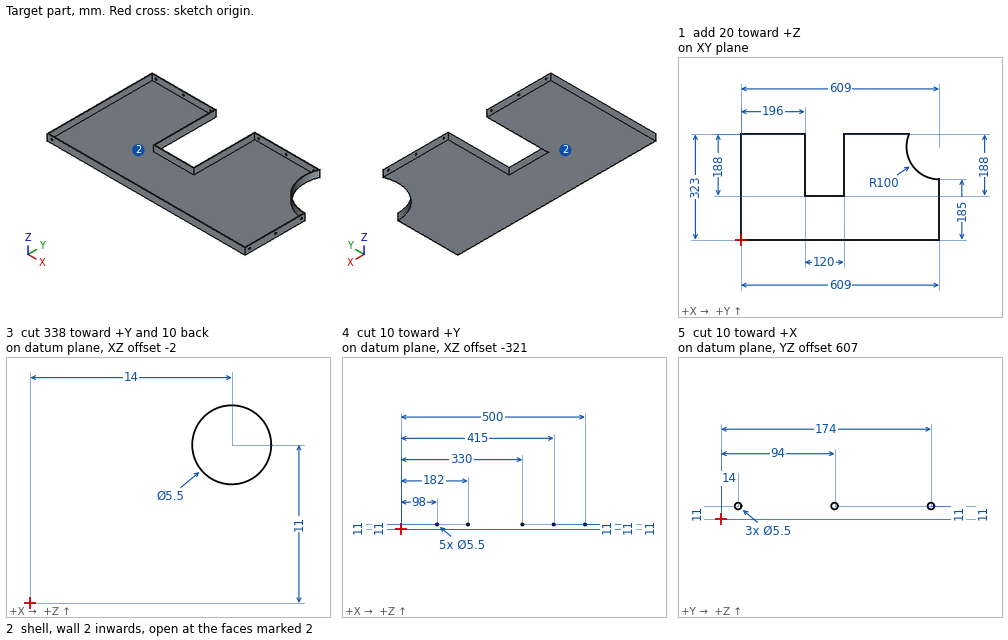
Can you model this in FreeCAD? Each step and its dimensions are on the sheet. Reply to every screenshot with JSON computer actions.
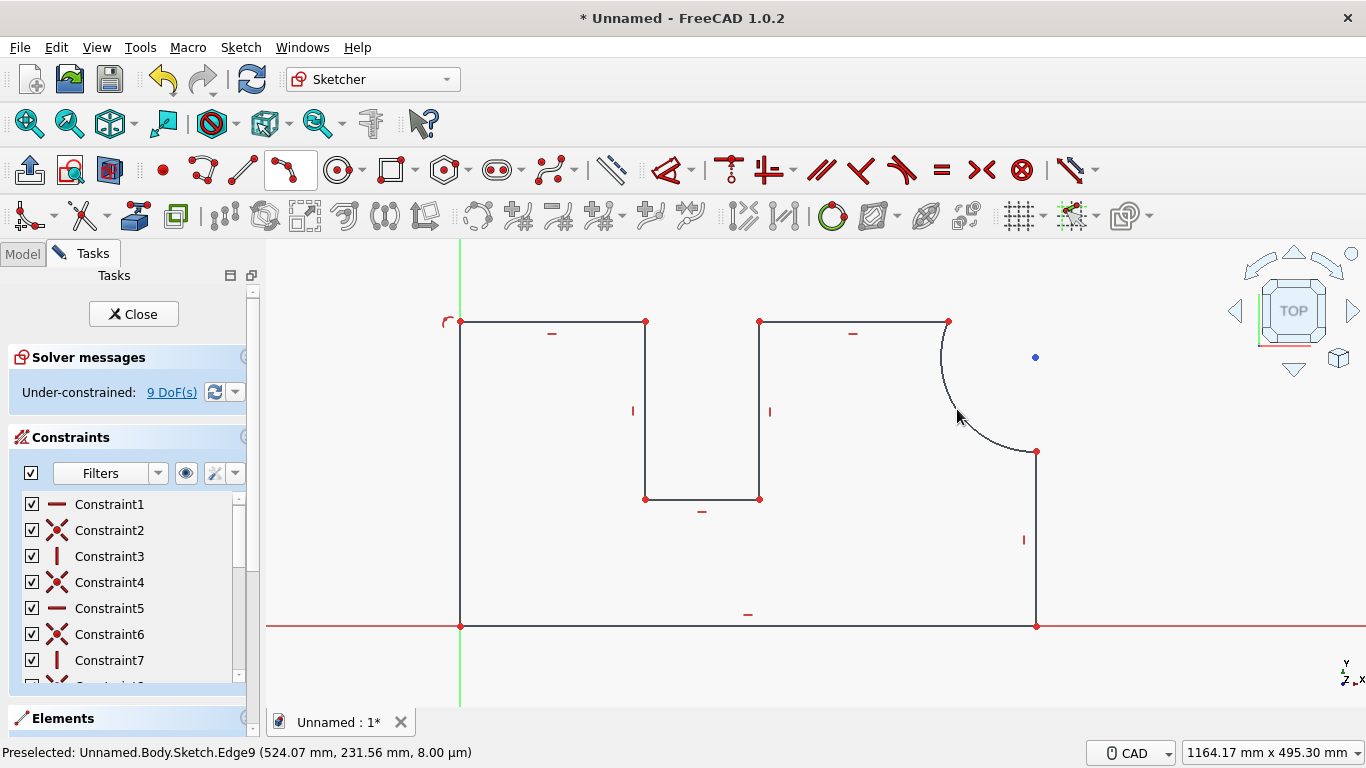
{"action": "left_click", "coordinate": [943, 377]}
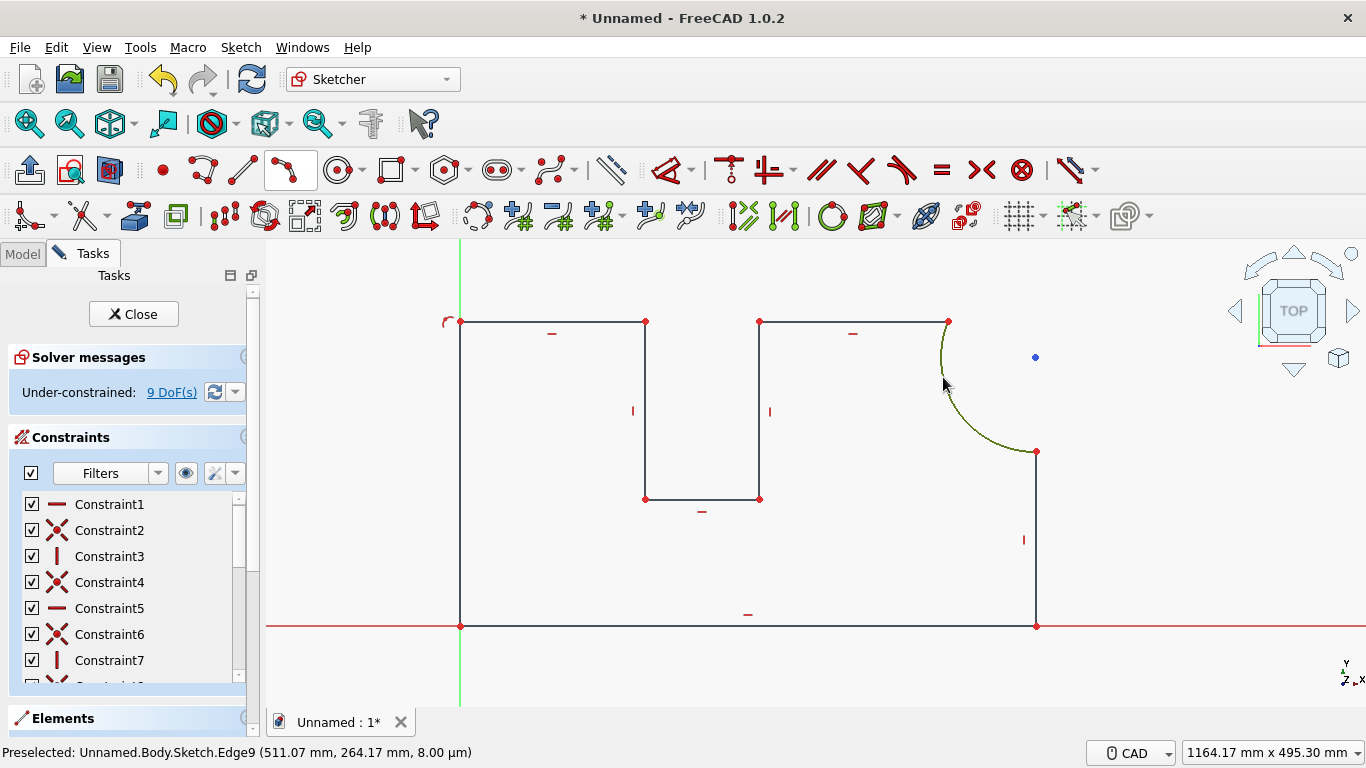
{"action": "key", "text": "k r"}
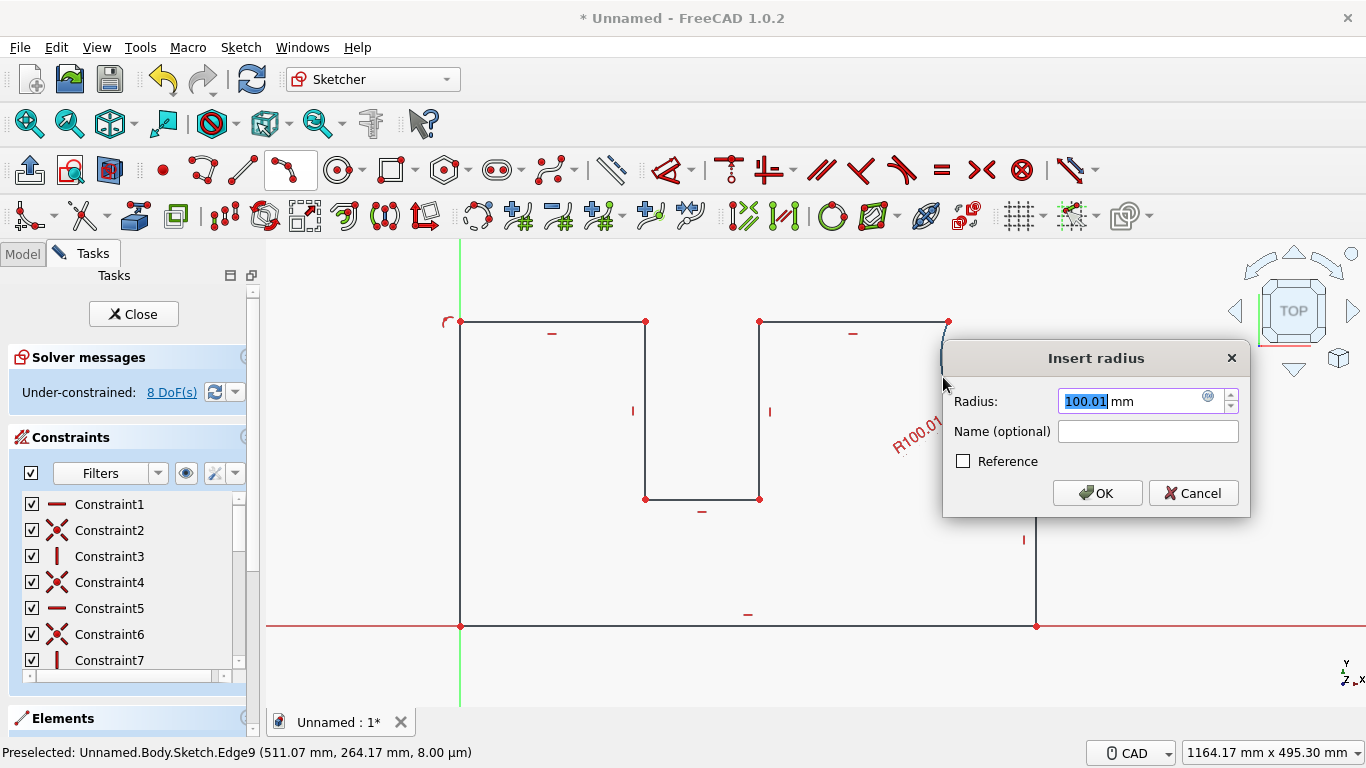
{"action": "type", "text": "100"}
{"action": "key", "text": "Return"}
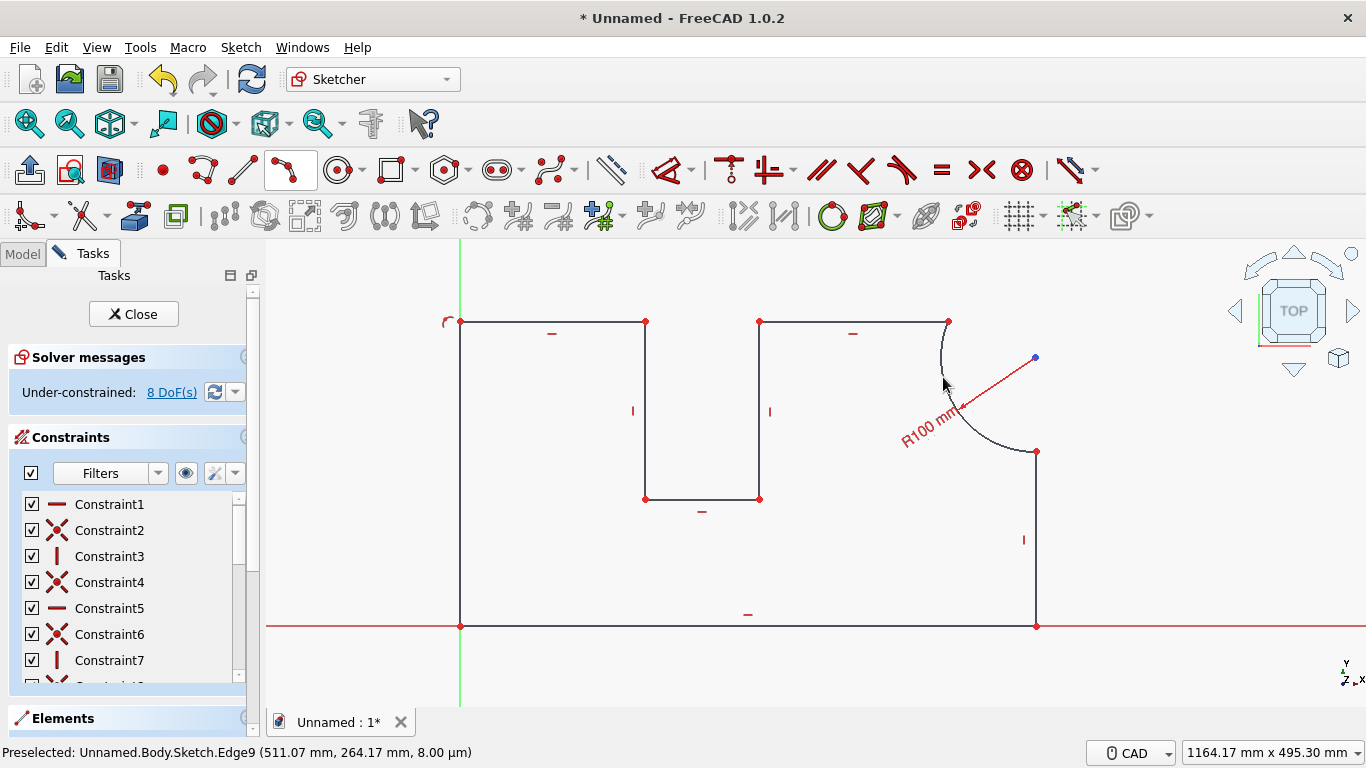
{"action": "left_click", "coordinate": [759, 375]}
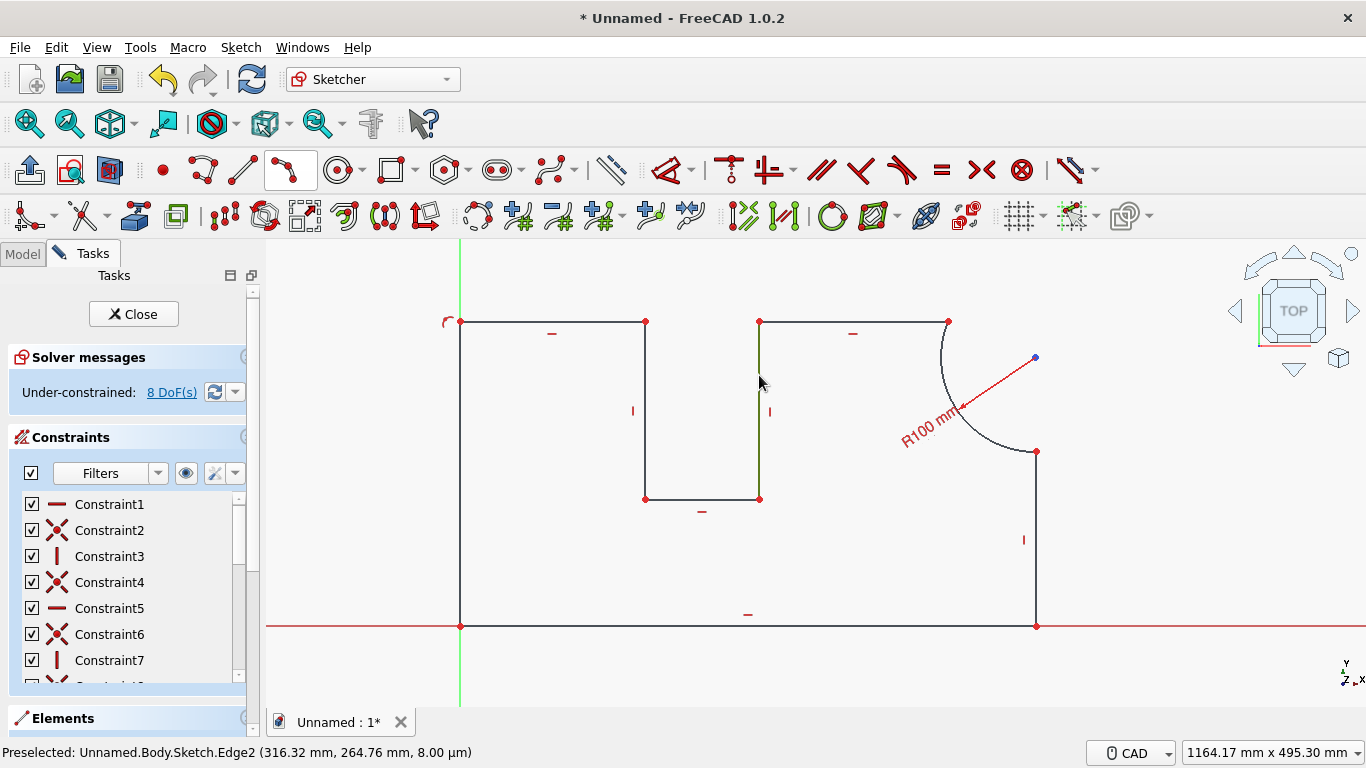
{"action": "key", "text": "i"}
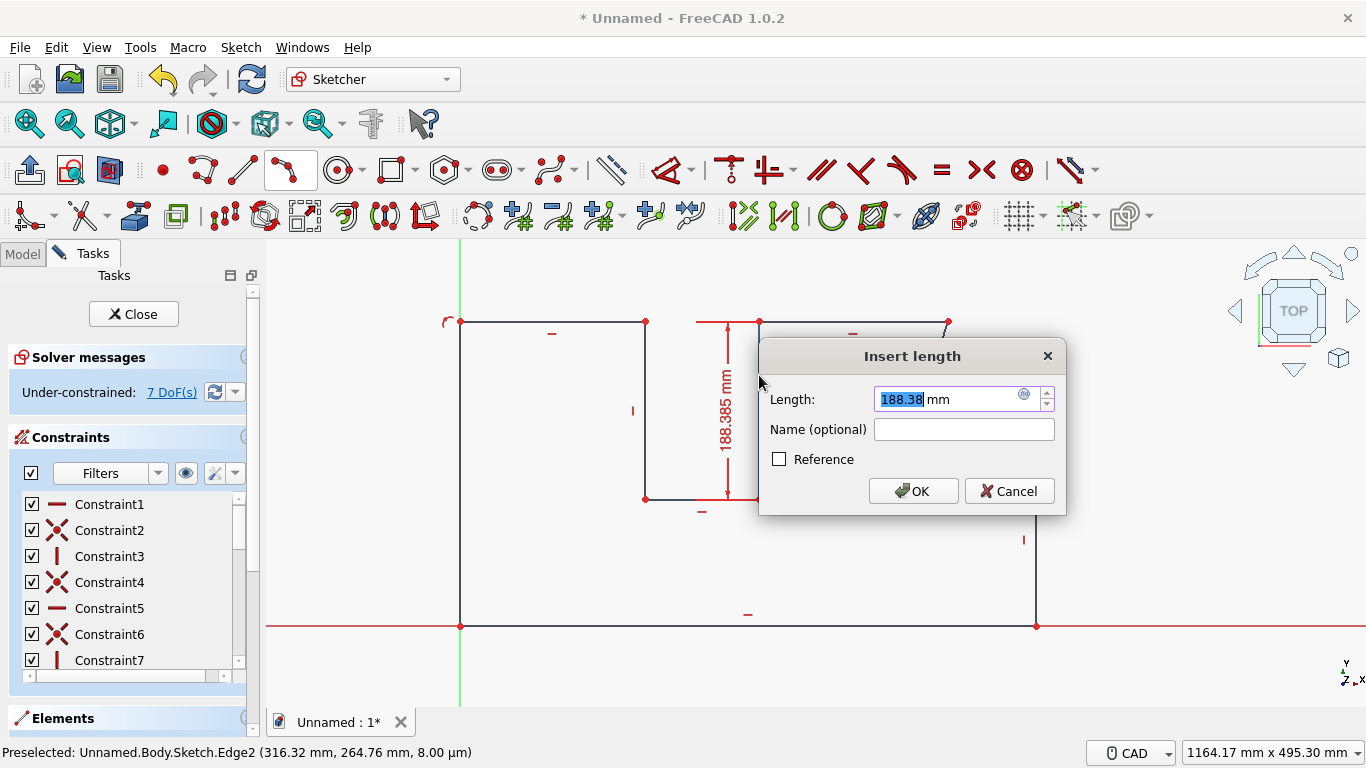
{"action": "type", "text": "188"}
{"action": "key", "text": "Return"}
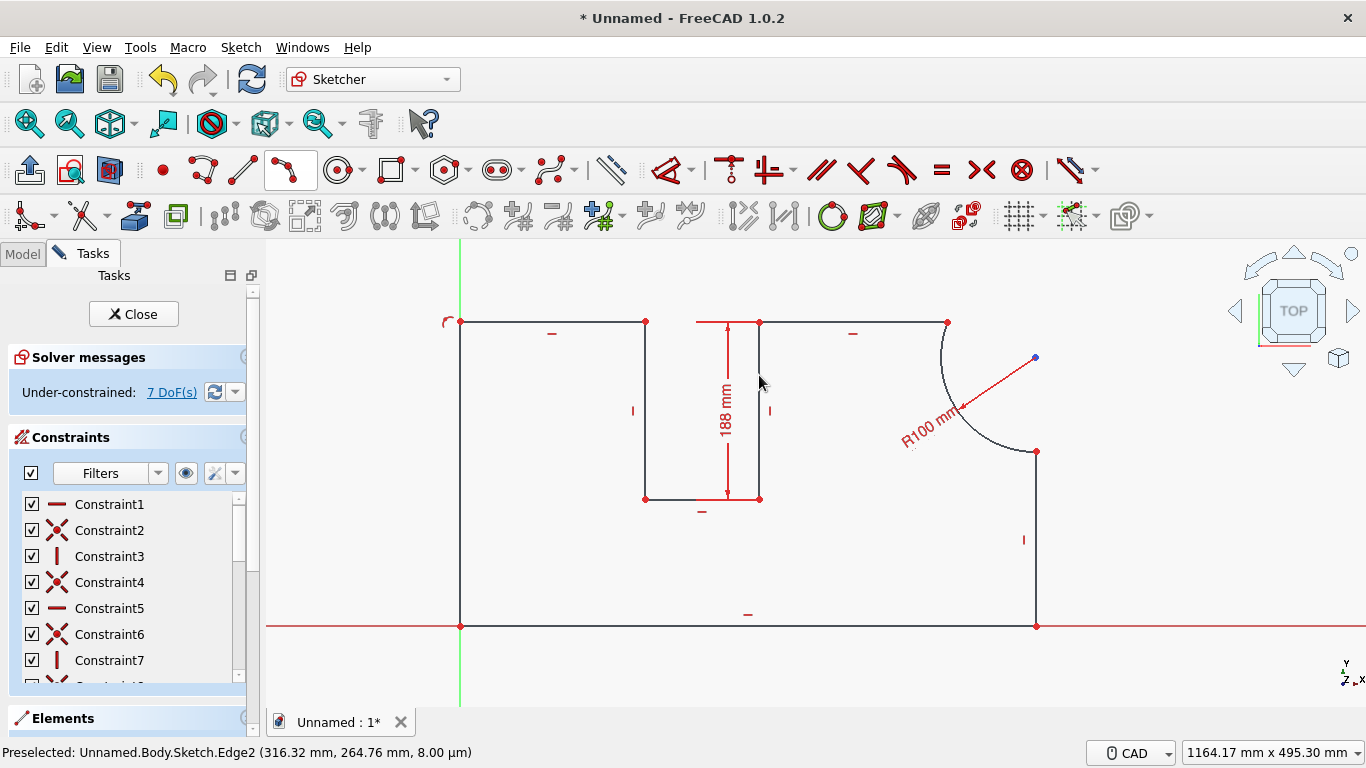
{"action": "left_click", "coordinate": [725, 500]}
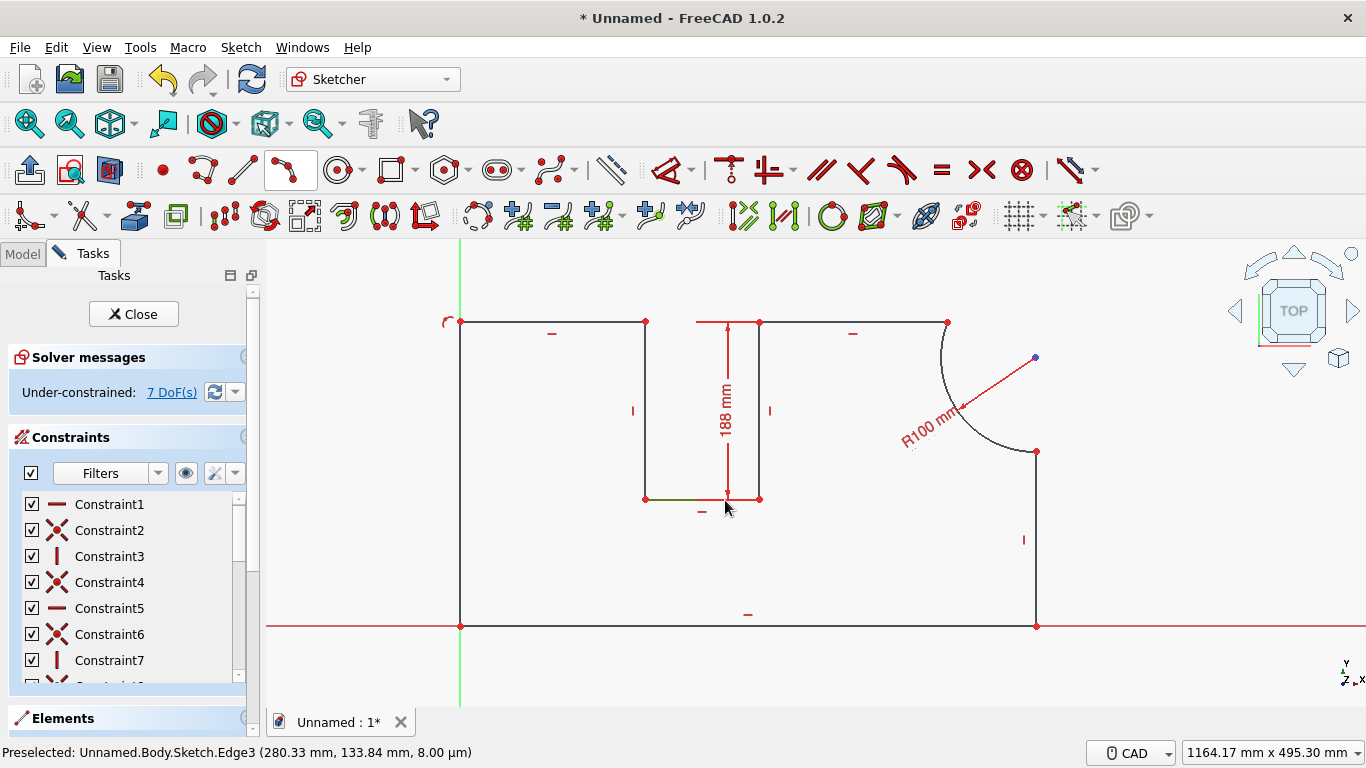
{"action": "key", "text": "l"}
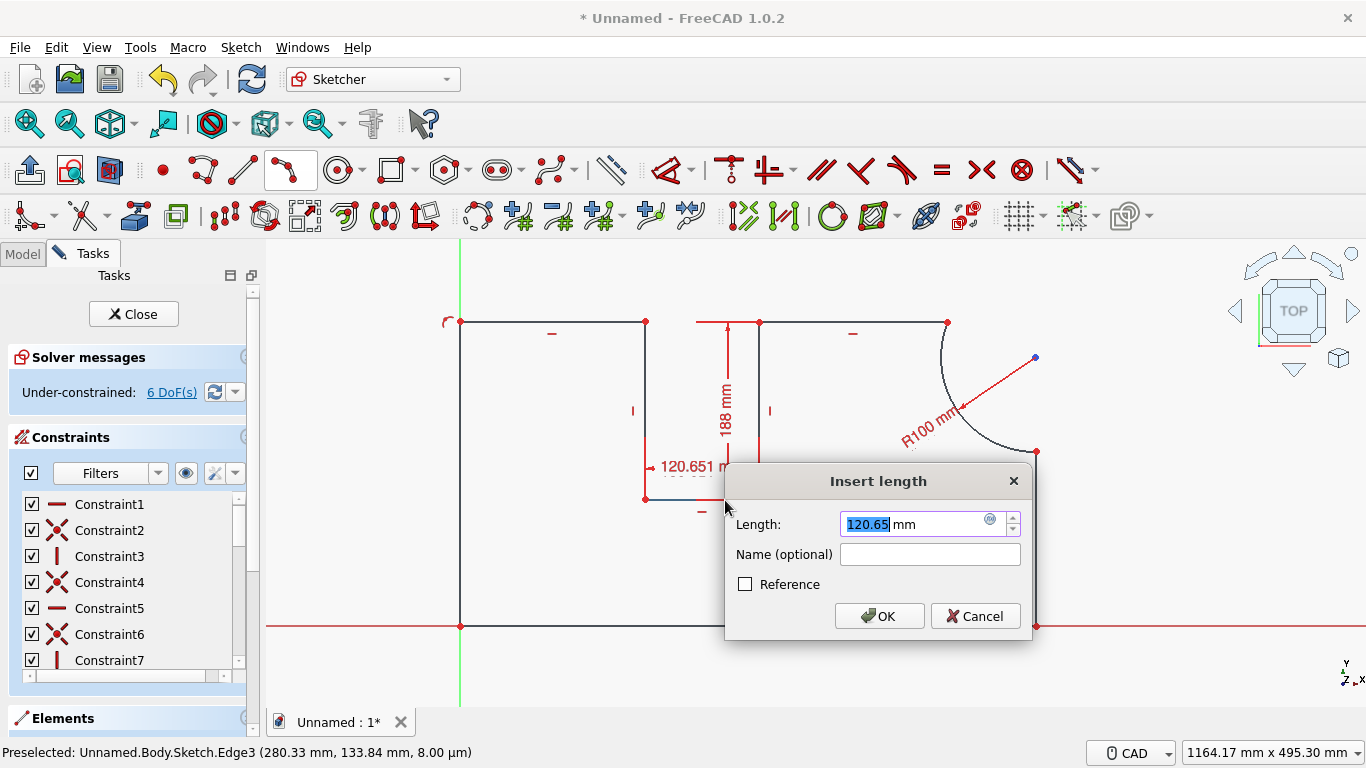
{"action": "type", "text": "120"}
{"action": "key", "text": "Return"}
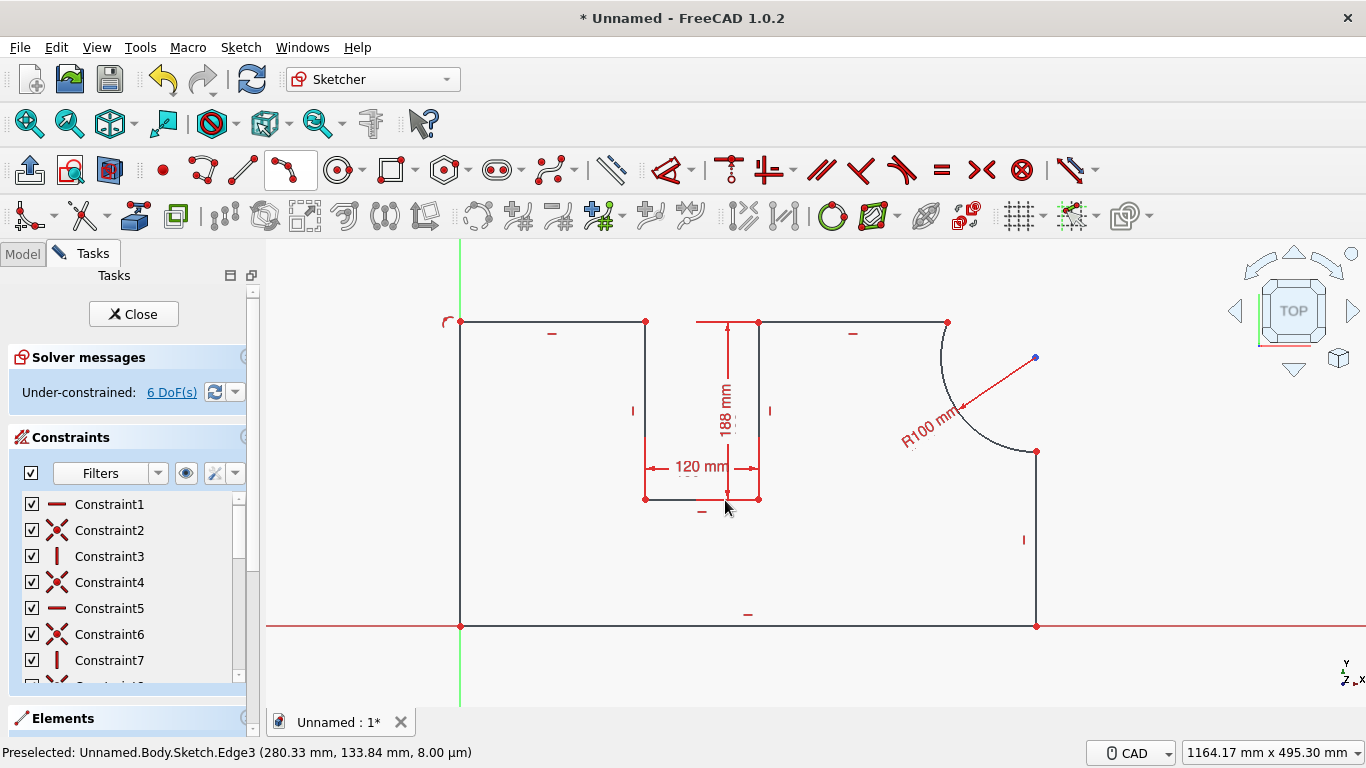
{"action": "left_click", "coordinate": [645, 446]}